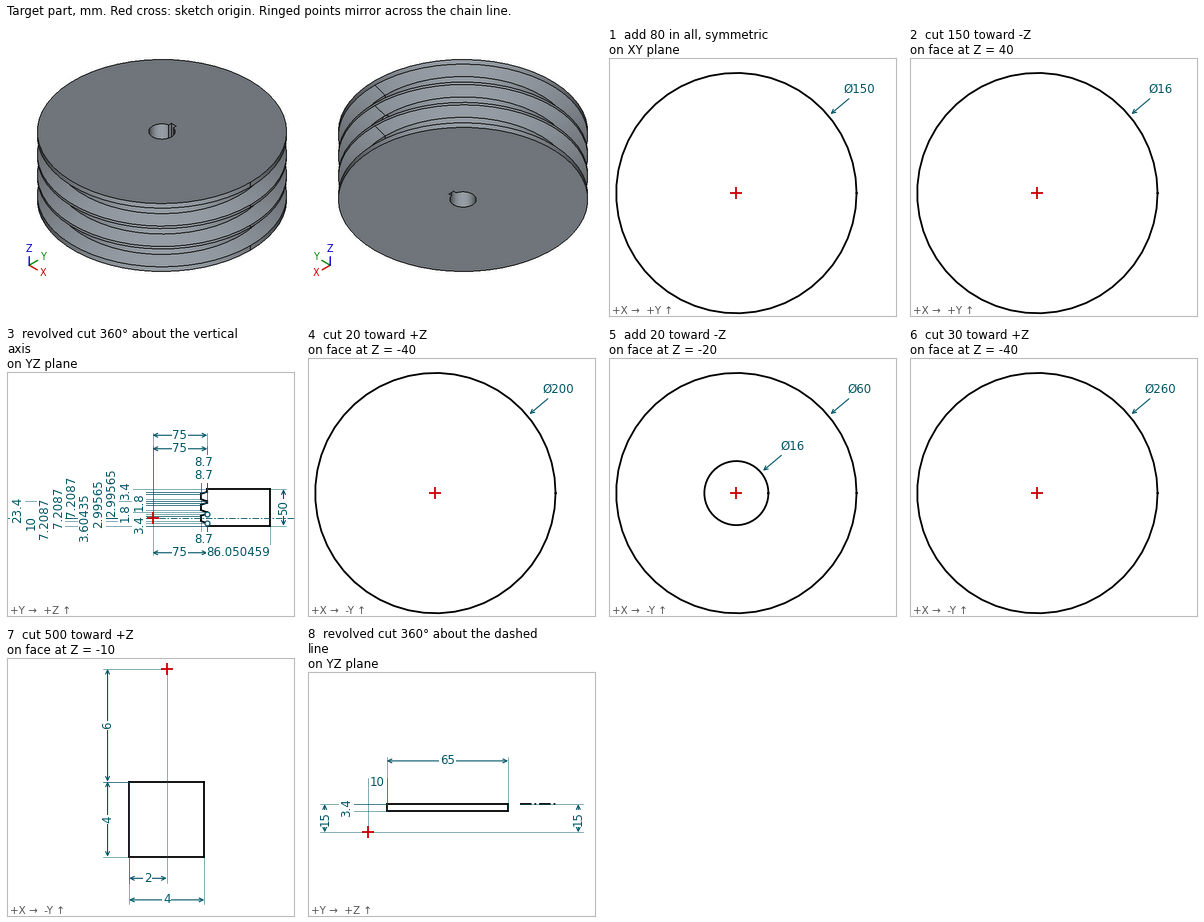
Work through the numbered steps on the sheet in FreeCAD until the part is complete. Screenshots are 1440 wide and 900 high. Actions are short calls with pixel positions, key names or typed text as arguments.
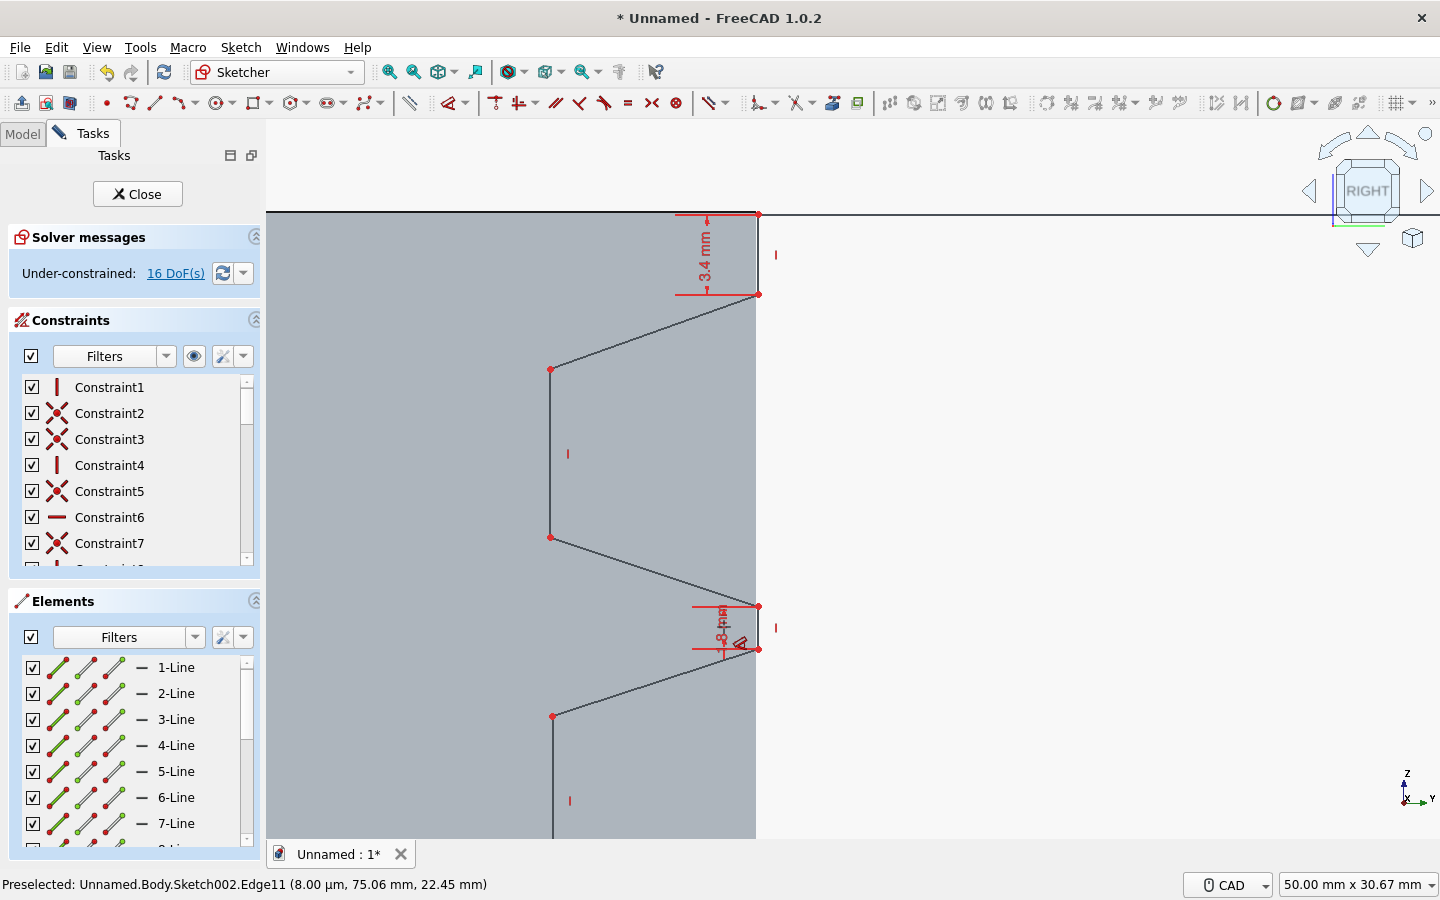
scroll(759, 398, down, 8)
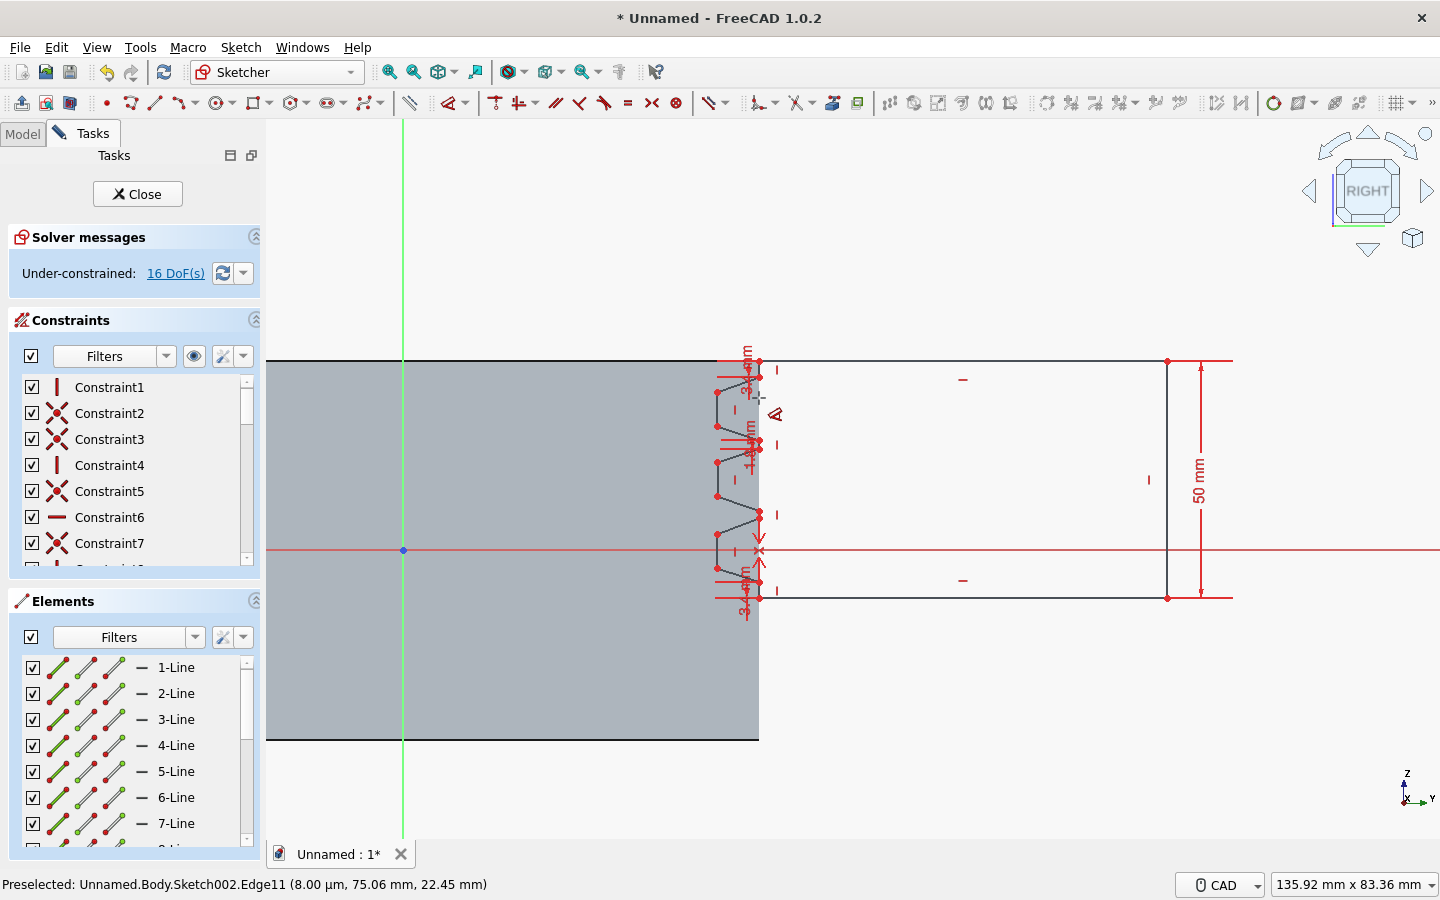
scroll(759, 513, up, 10)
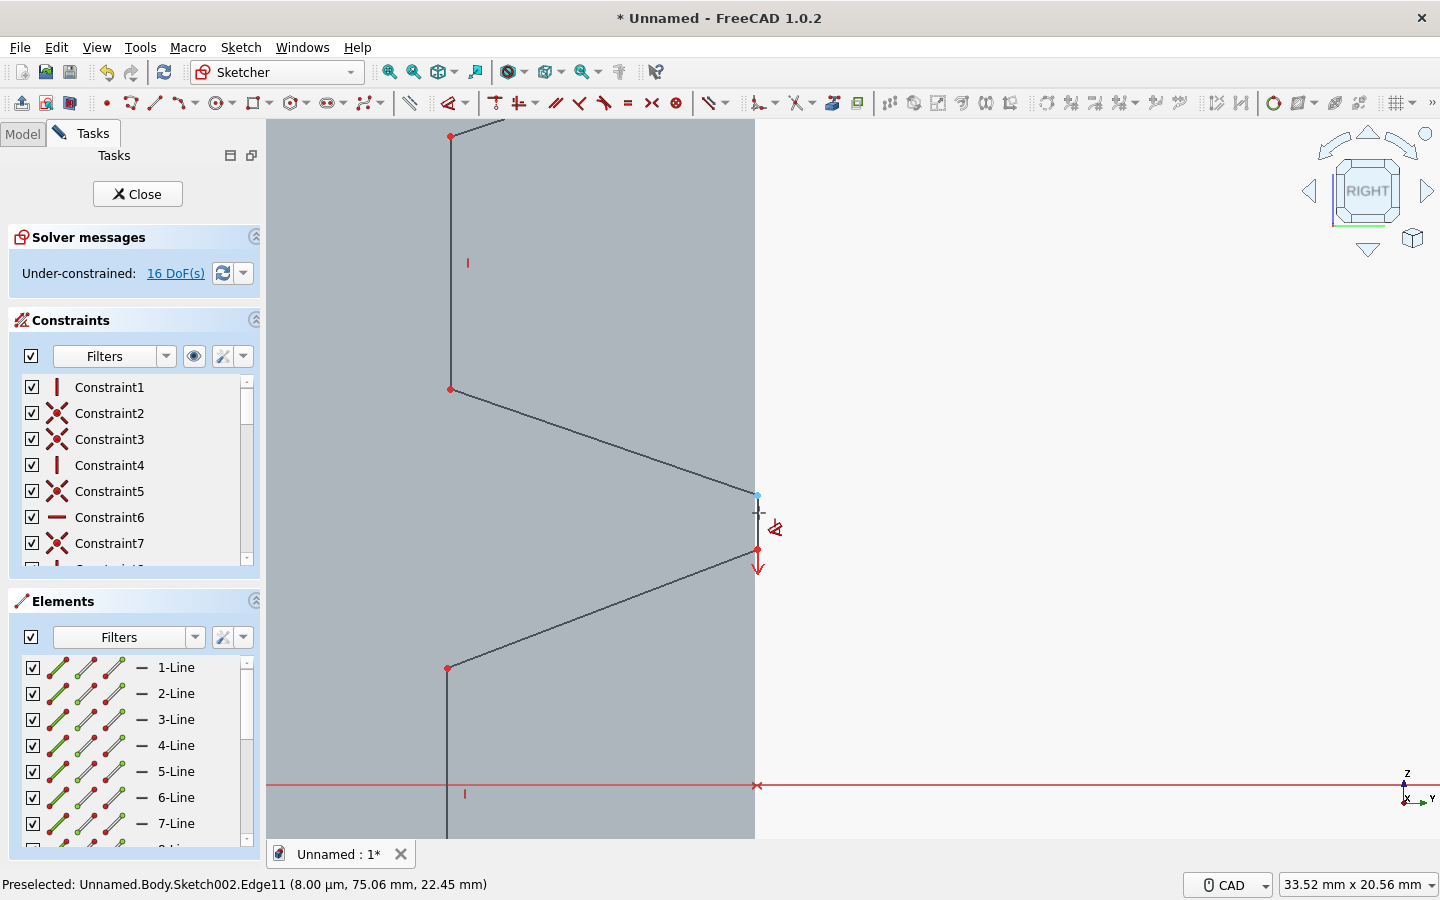
click(758, 512)
click(724, 522)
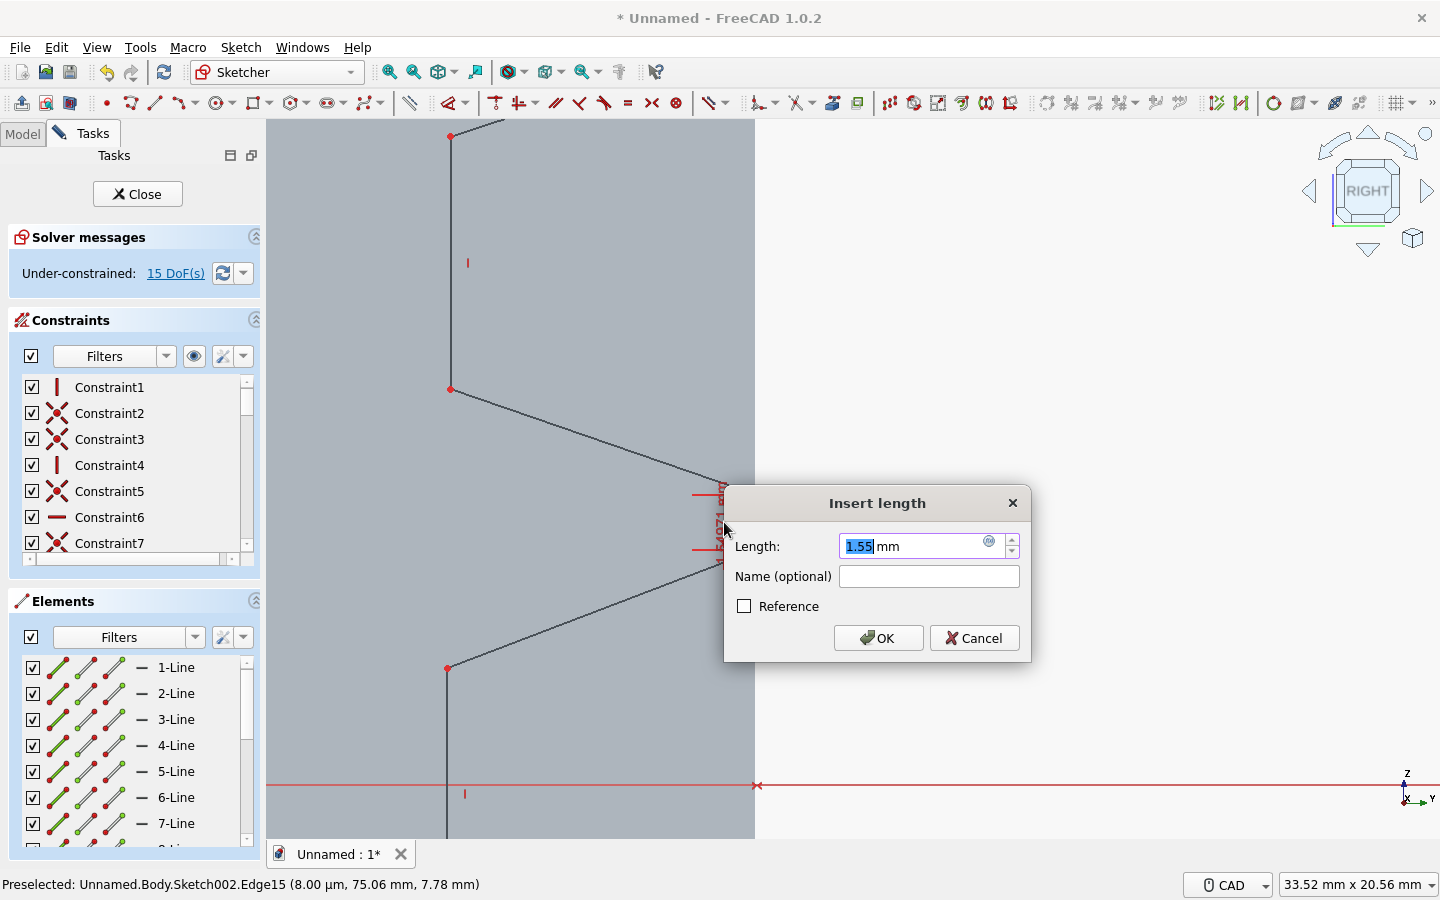
text(1.8)
key(Return)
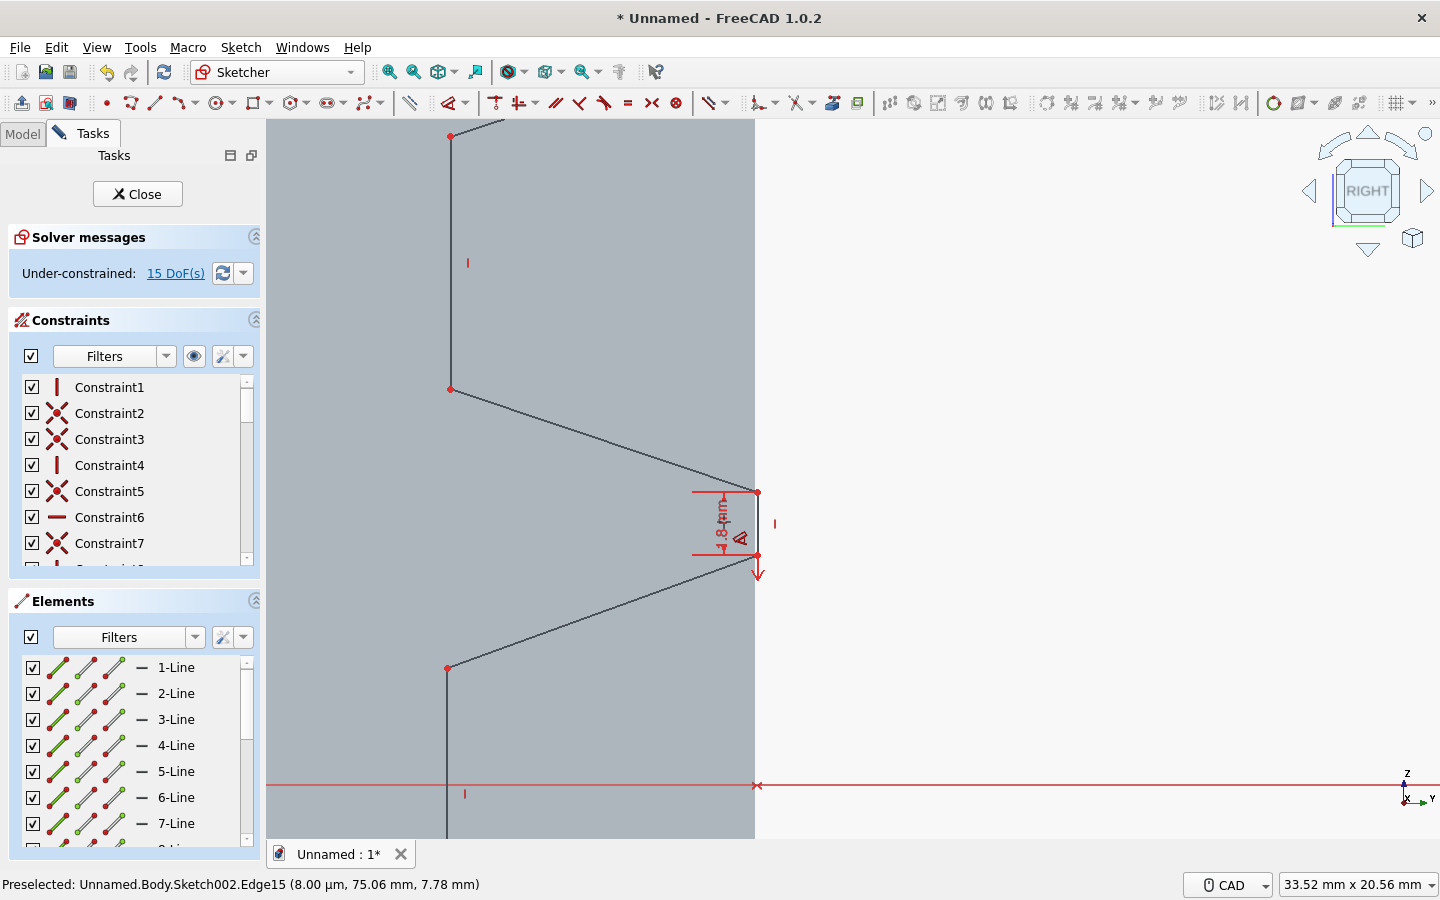
scroll(759, 513, down, 10)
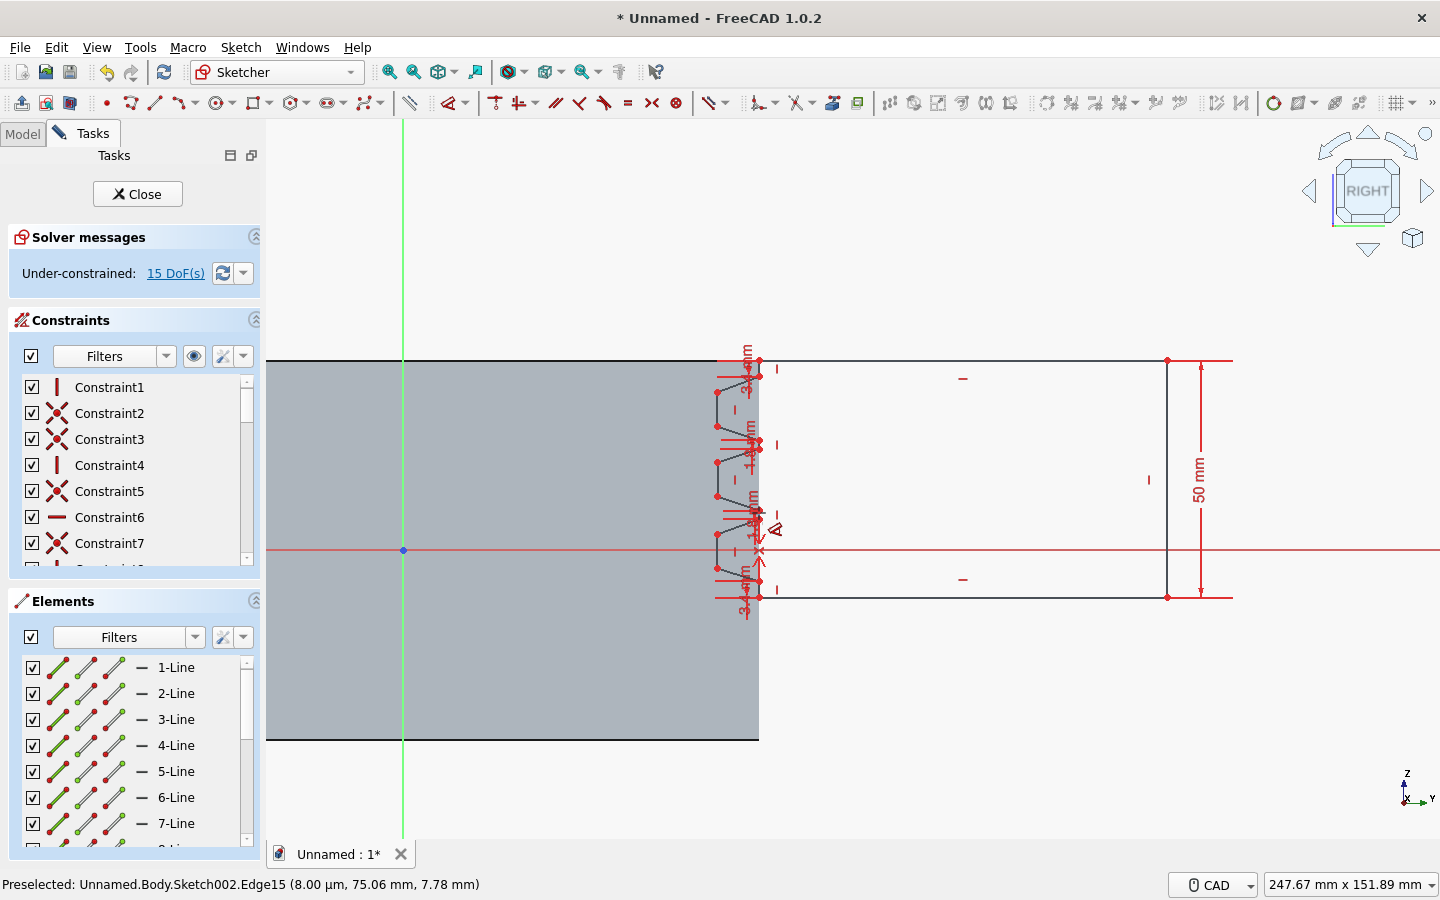
click(759, 581)
click(581, 615)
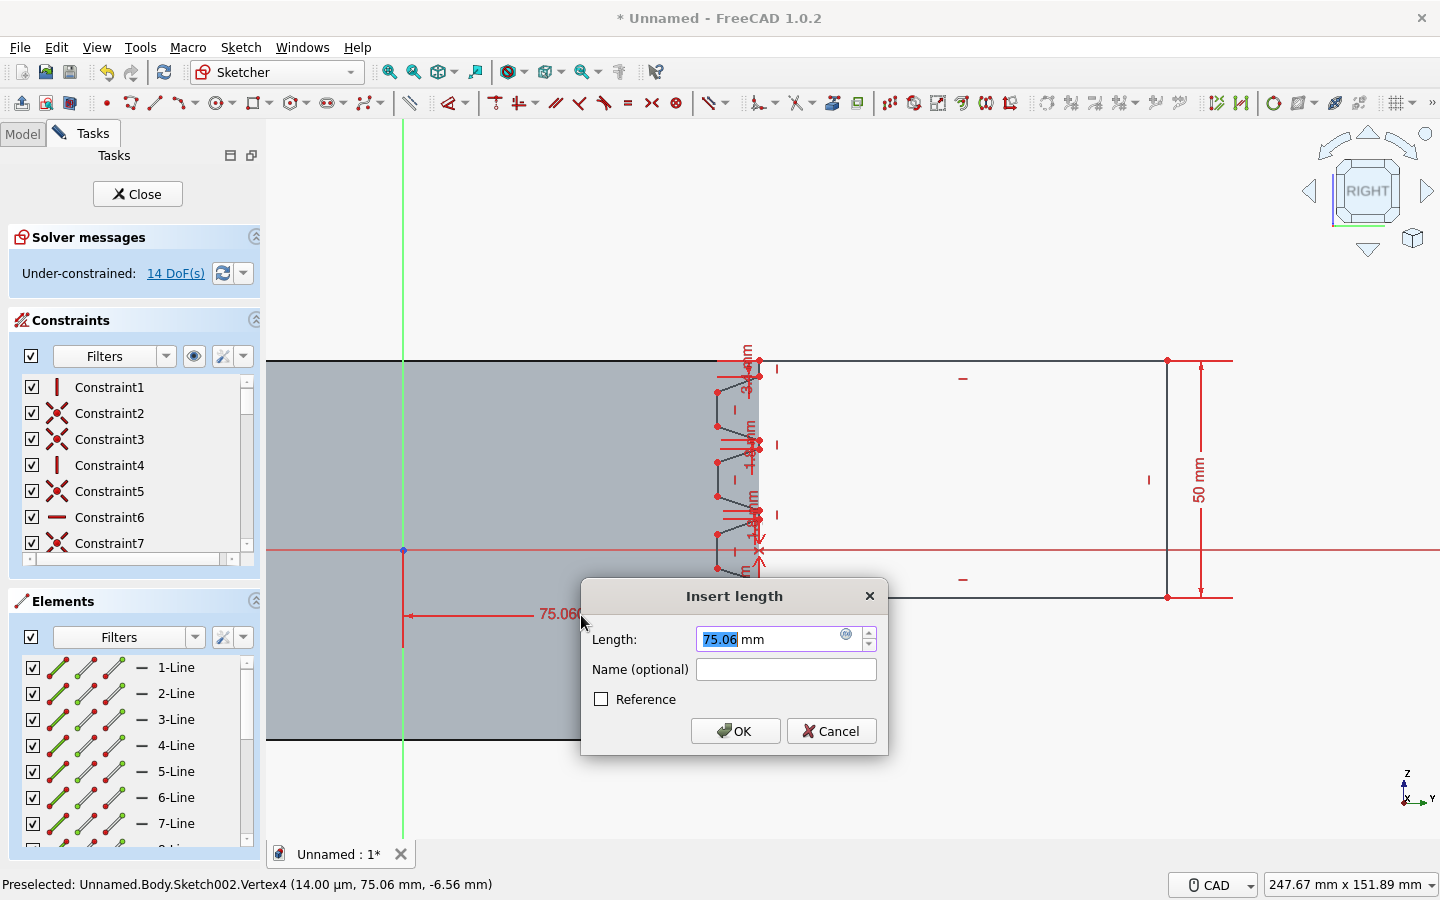
text(75)
key(Return)